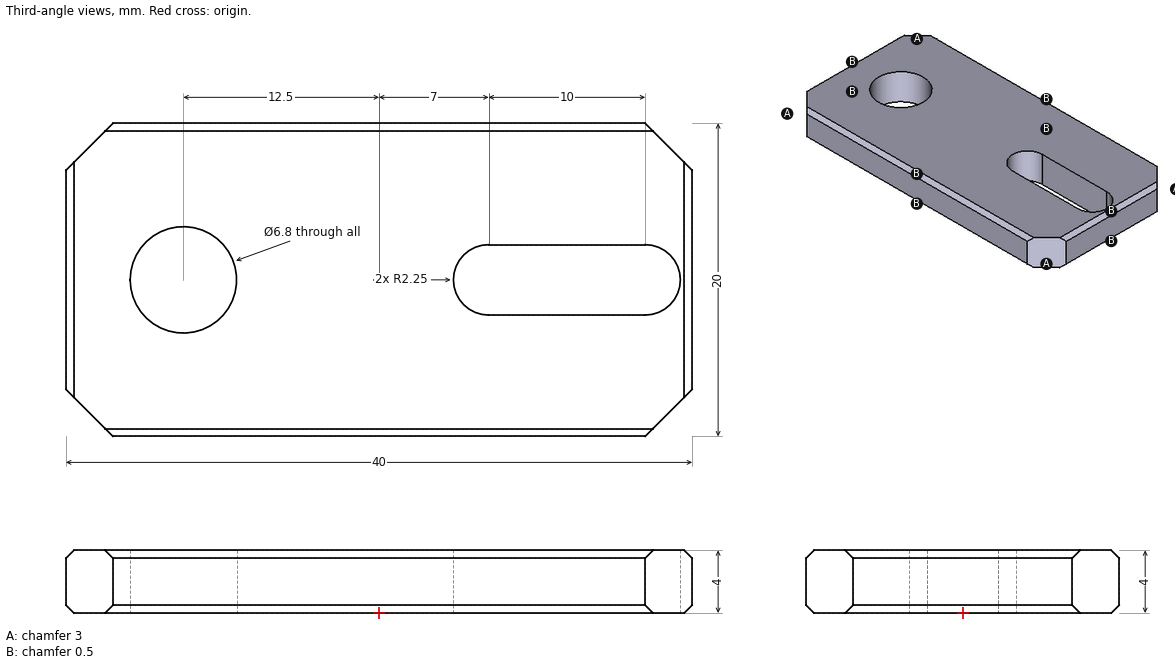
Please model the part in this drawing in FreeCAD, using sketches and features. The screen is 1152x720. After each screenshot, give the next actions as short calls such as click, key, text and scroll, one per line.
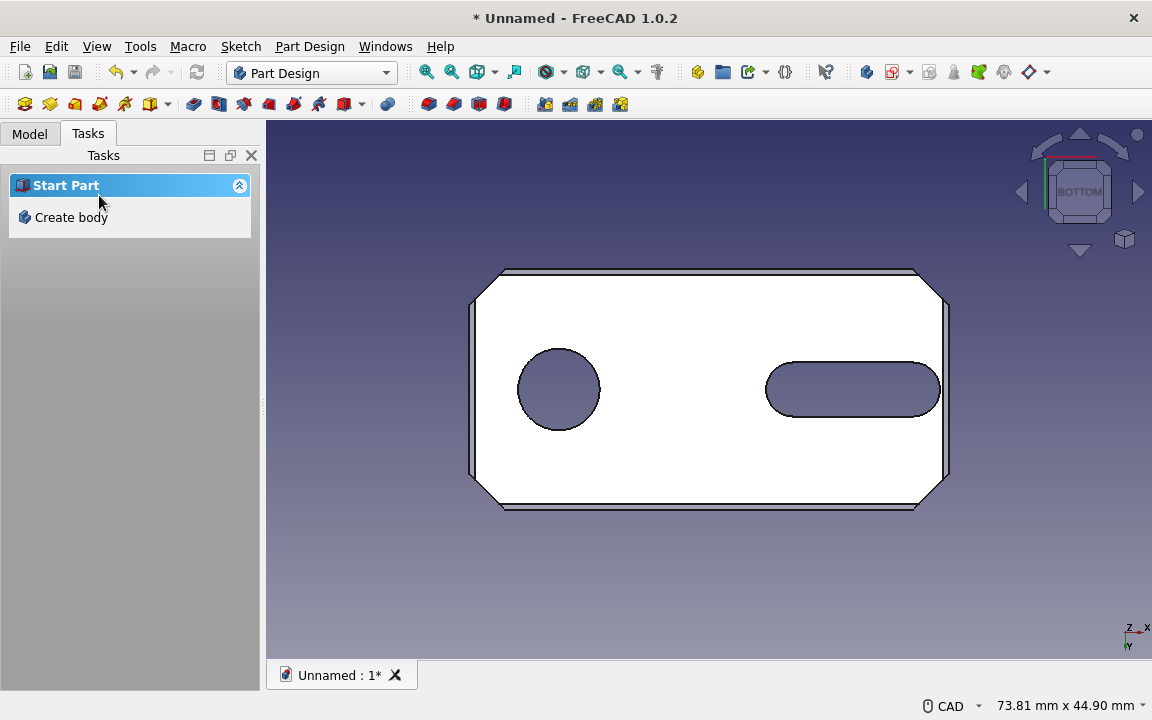
key(0)